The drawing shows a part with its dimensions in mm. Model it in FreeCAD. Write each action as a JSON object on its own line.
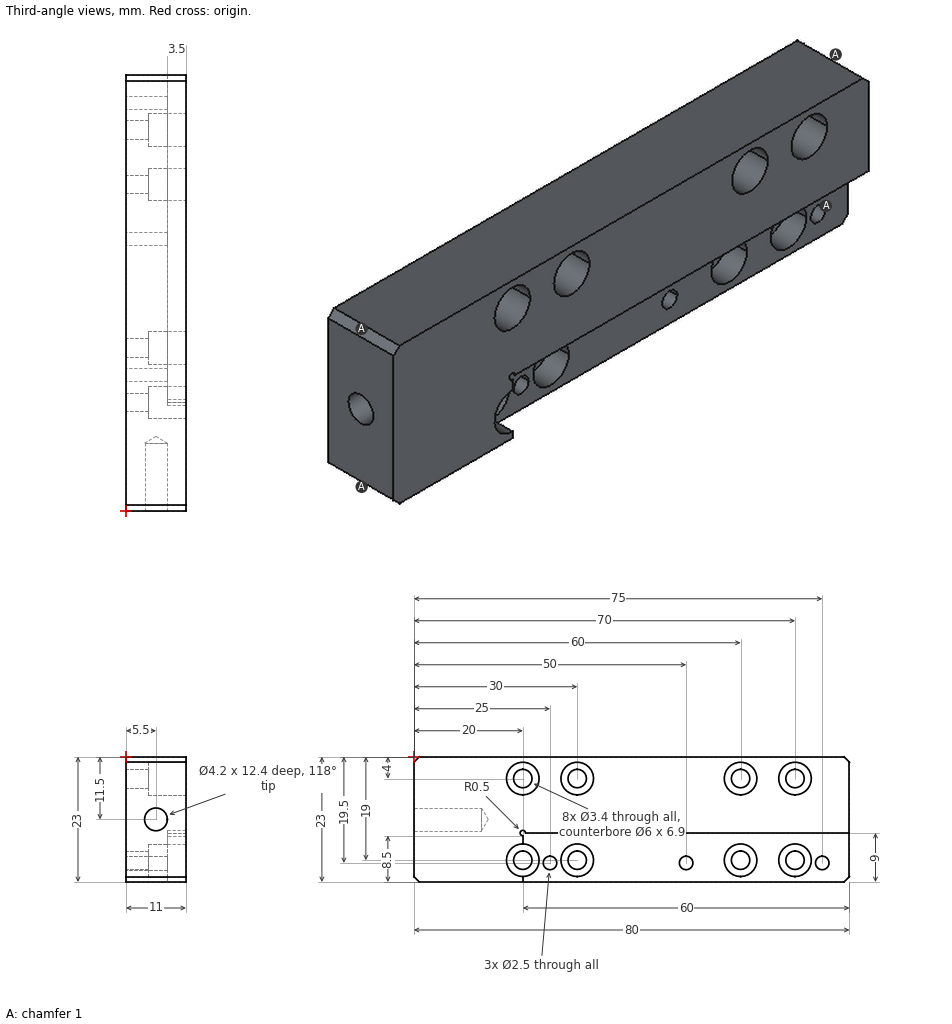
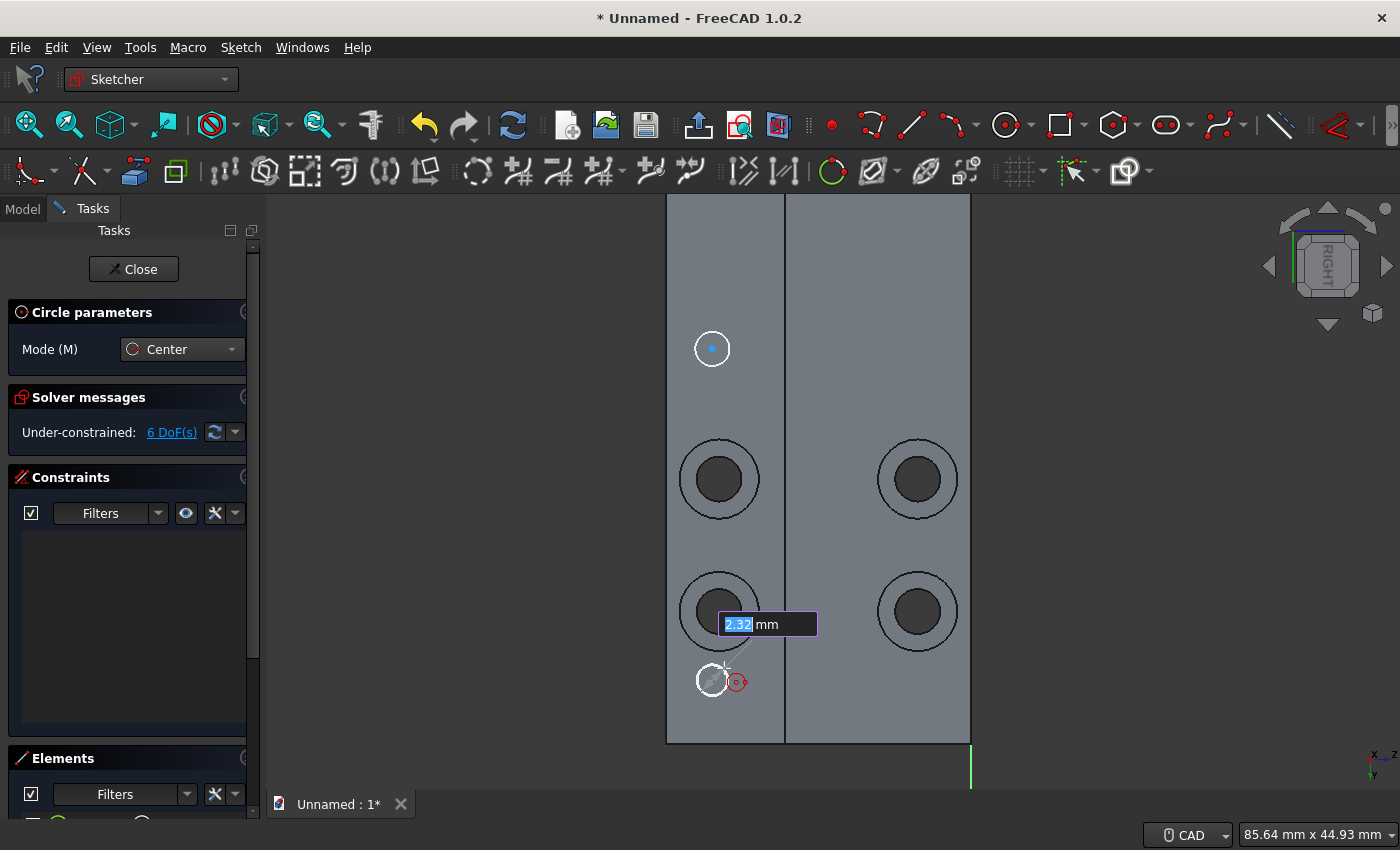
{"action": "left_click", "coordinate": [724, 666]}
{"action": "key", "text": "Escape"}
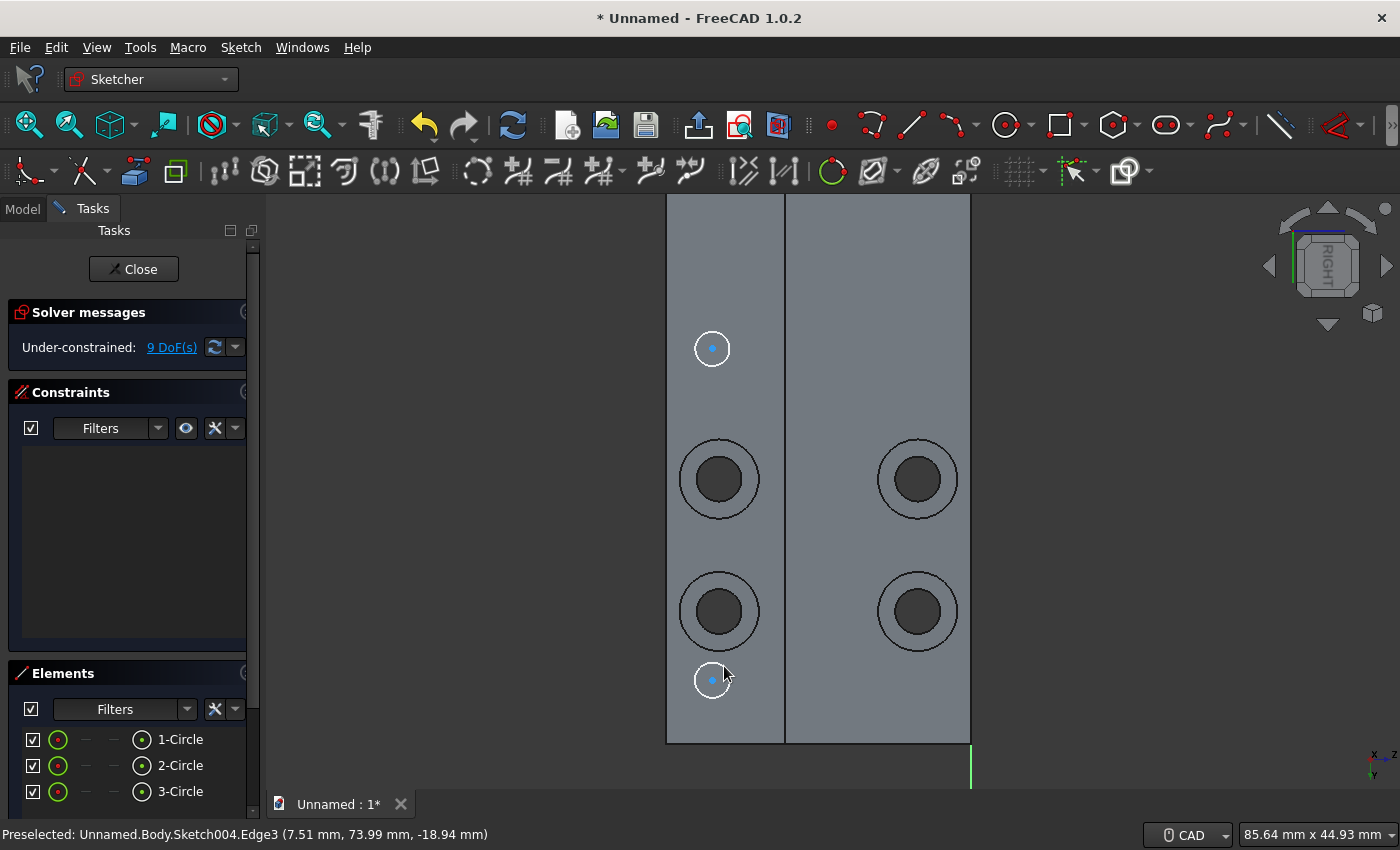
{"action": "scroll", "coordinate": [724, 667], "scroll_direction": "down", "scroll_amount": 5}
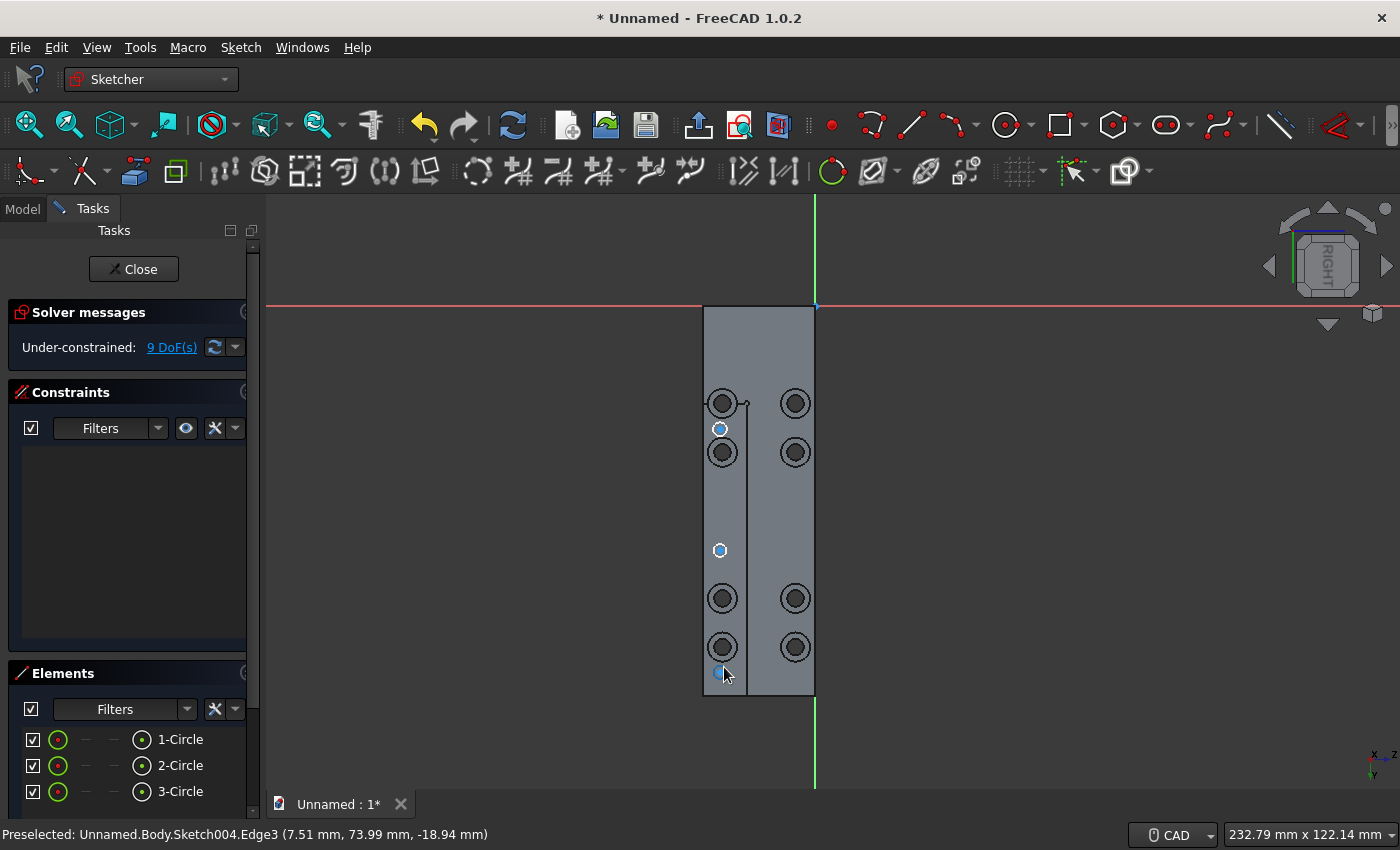
{"action": "scroll", "coordinate": [725, 424], "scroll_direction": "up", "scroll_amount": 4}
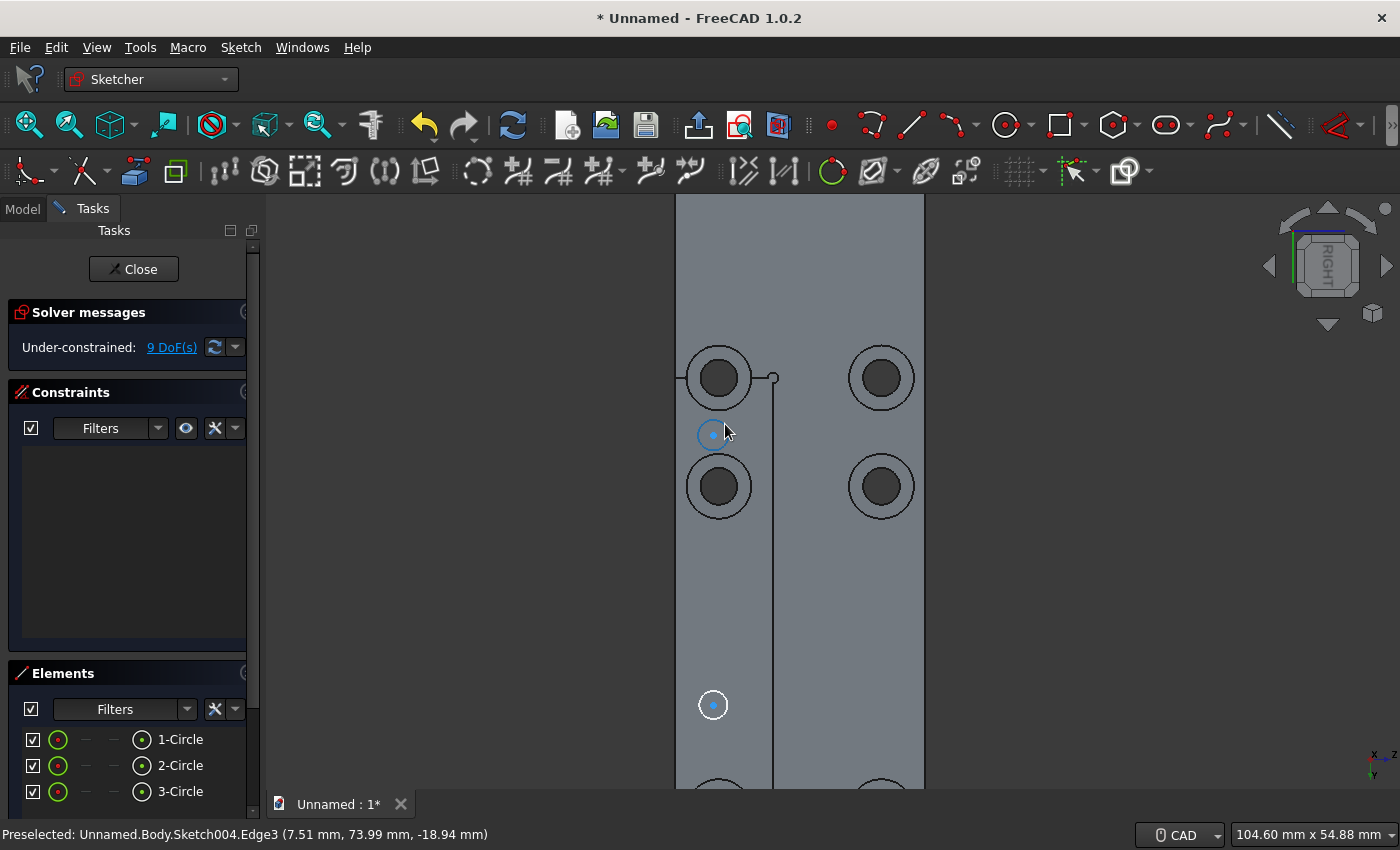
{"action": "left_click", "coordinate": [724, 424]}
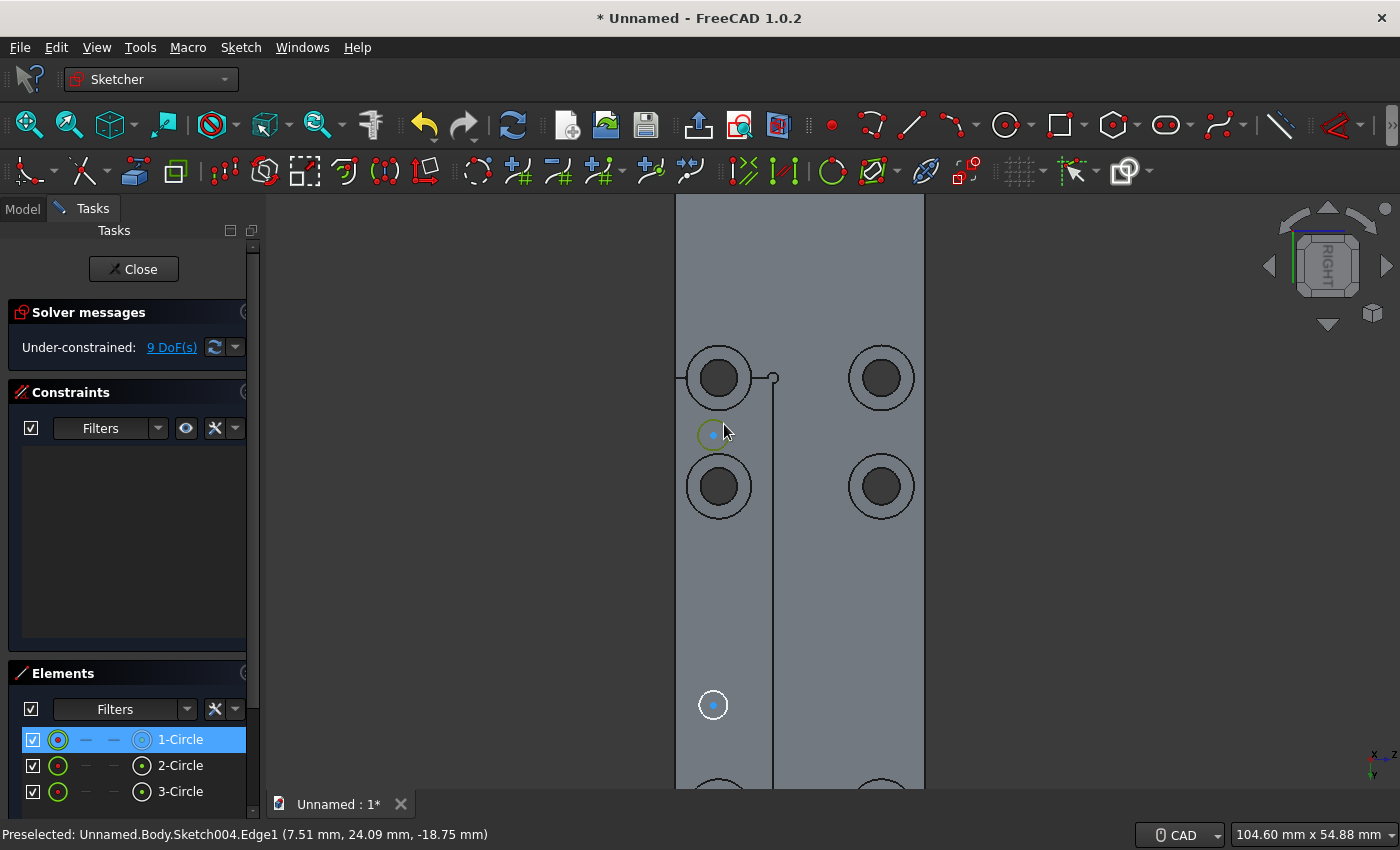
{"action": "left_click", "coordinate": [723, 695]}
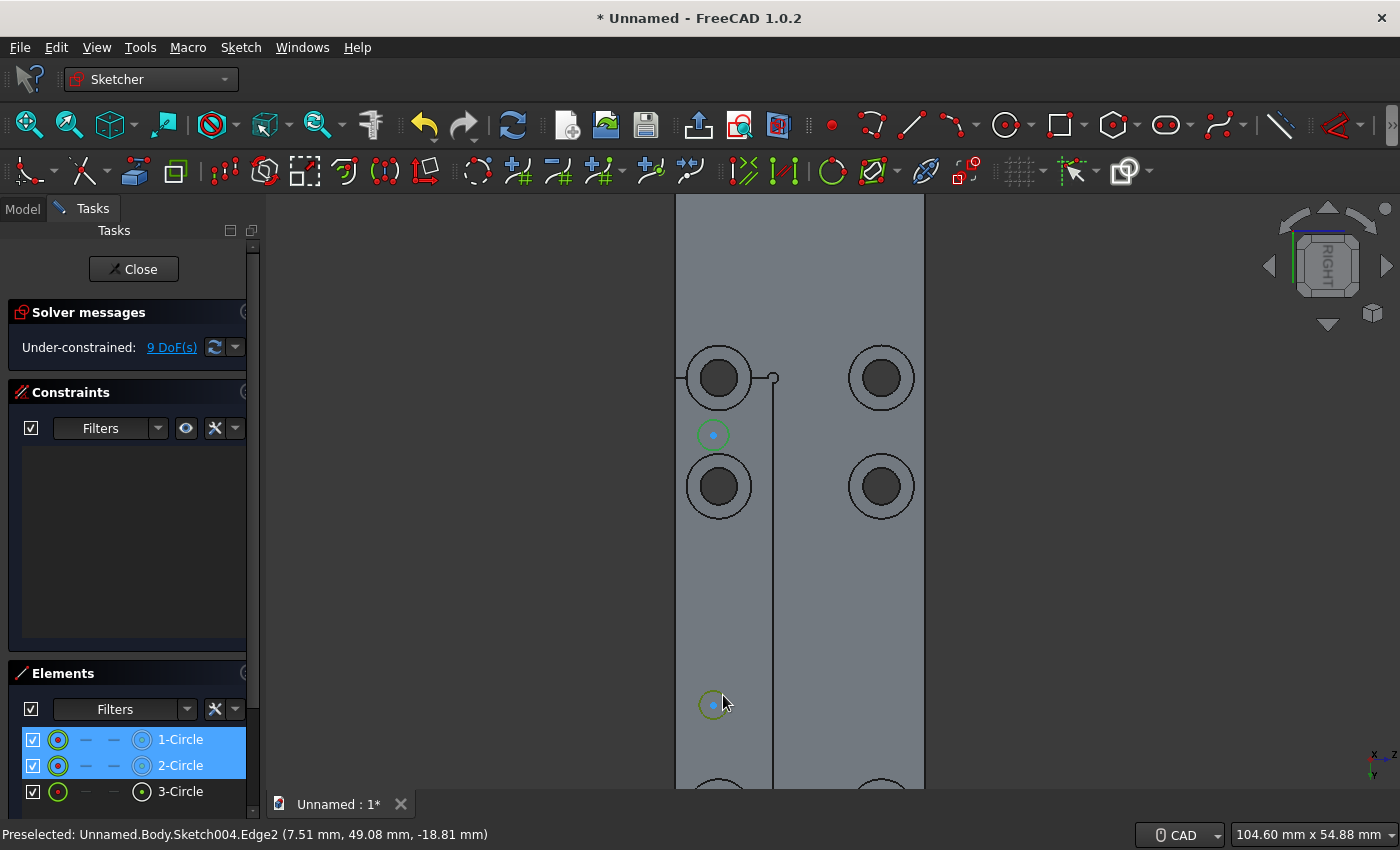
{"action": "scroll", "coordinate": [725, 424], "scroll_direction": "down", "scroll_amount": 4}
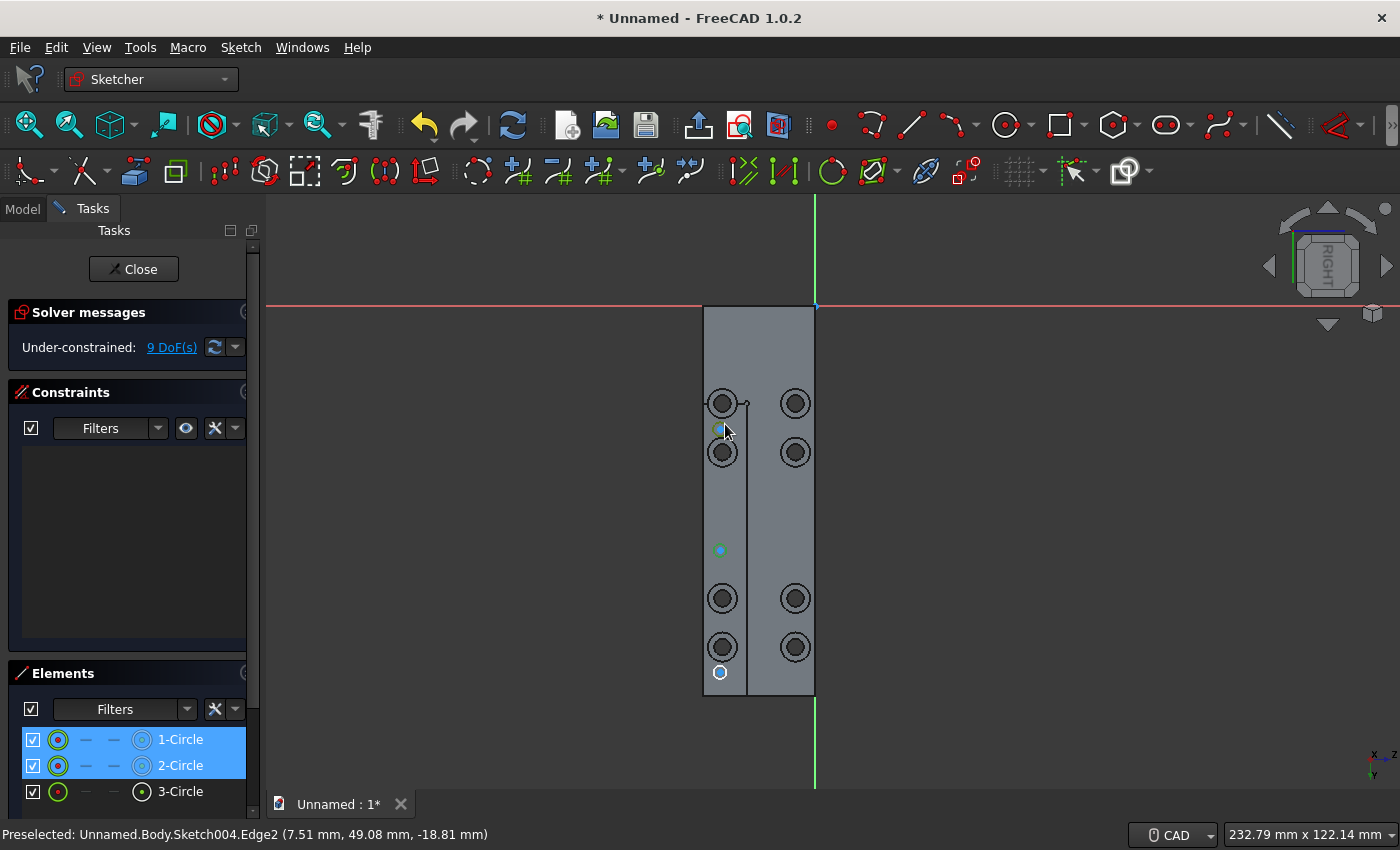
{"action": "scroll", "coordinate": [725, 668], "scroll_direction": "up", "scroll_amount": 4}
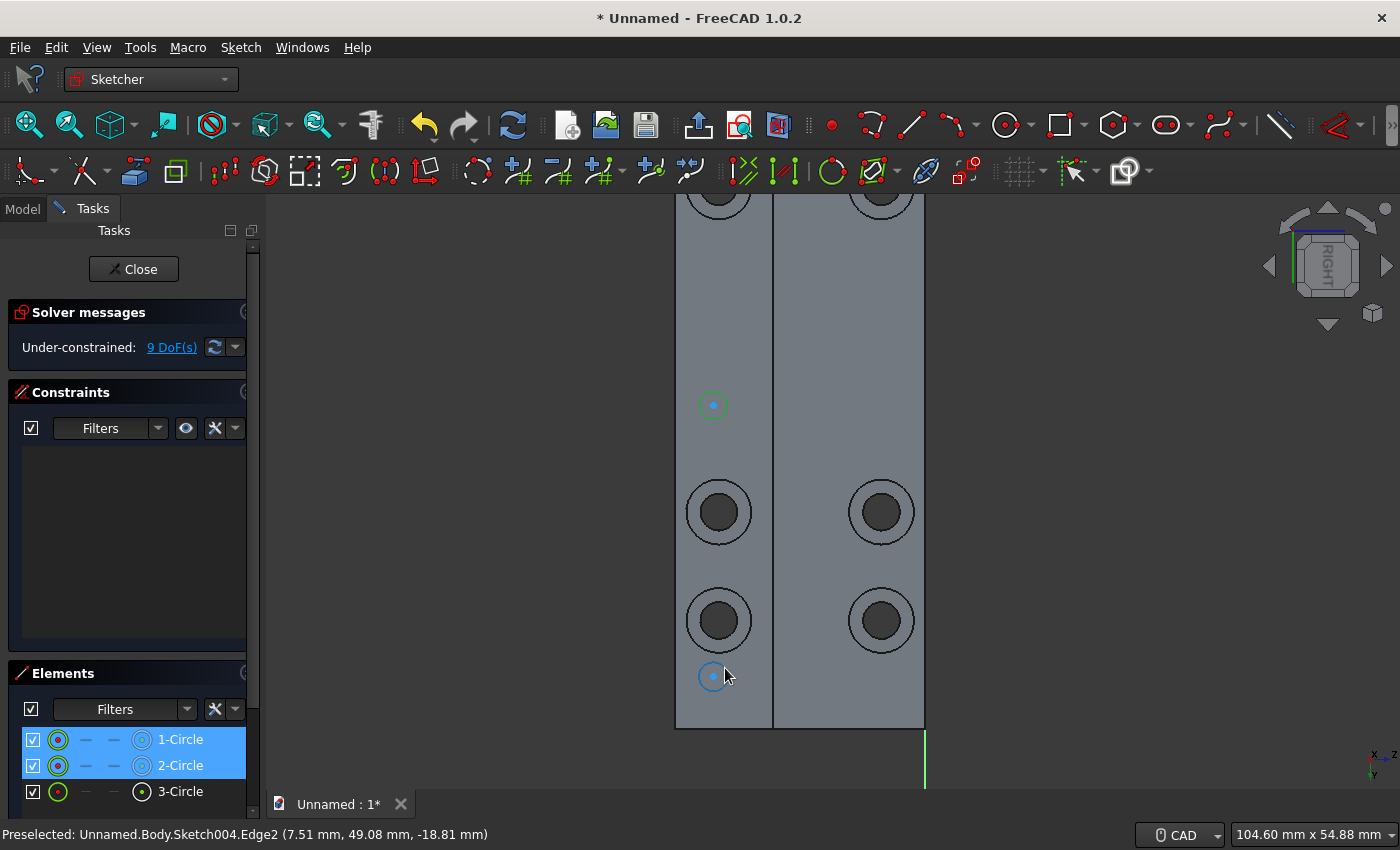
{"action": "left_click", "coordinate": [724, 667]}